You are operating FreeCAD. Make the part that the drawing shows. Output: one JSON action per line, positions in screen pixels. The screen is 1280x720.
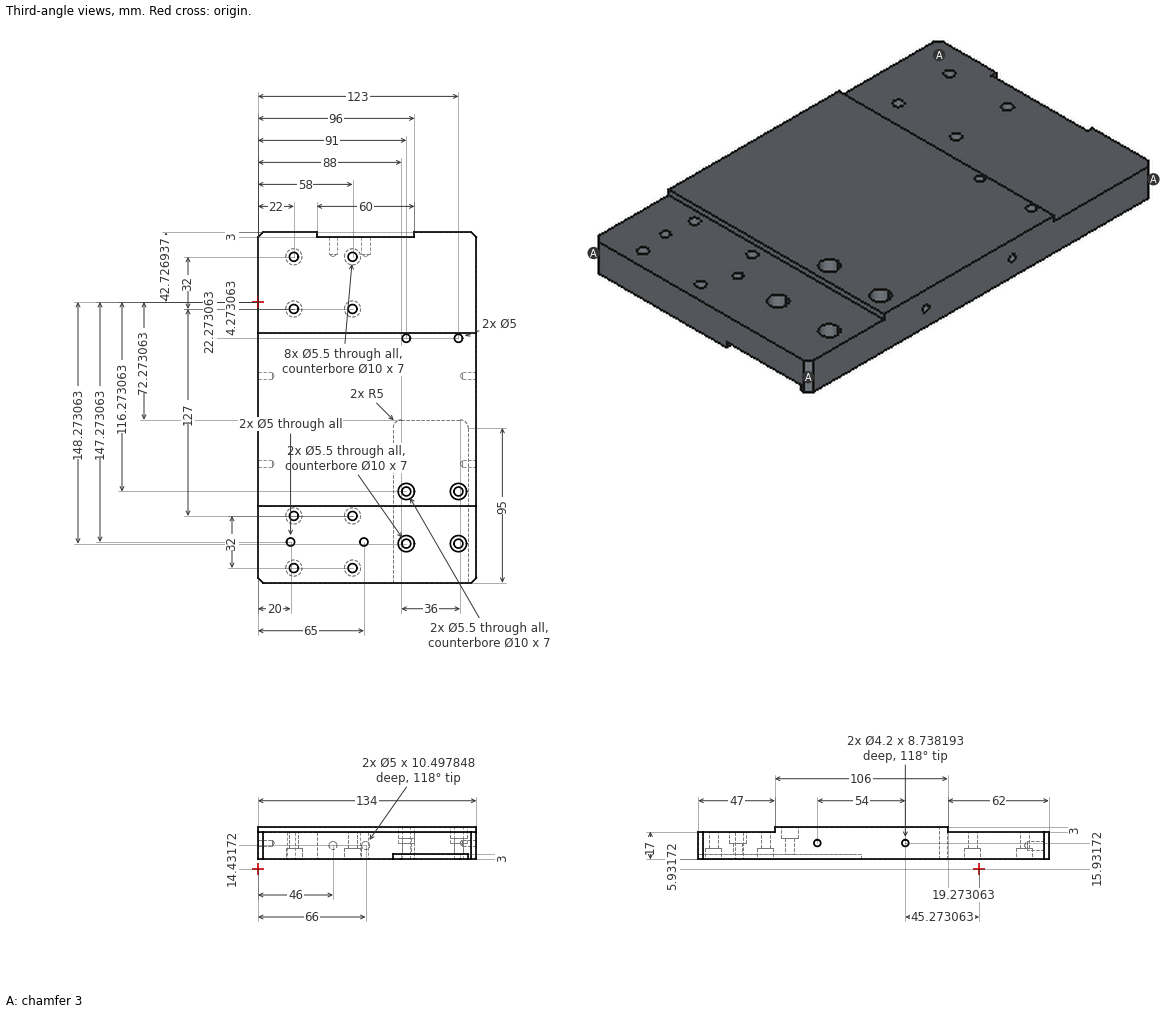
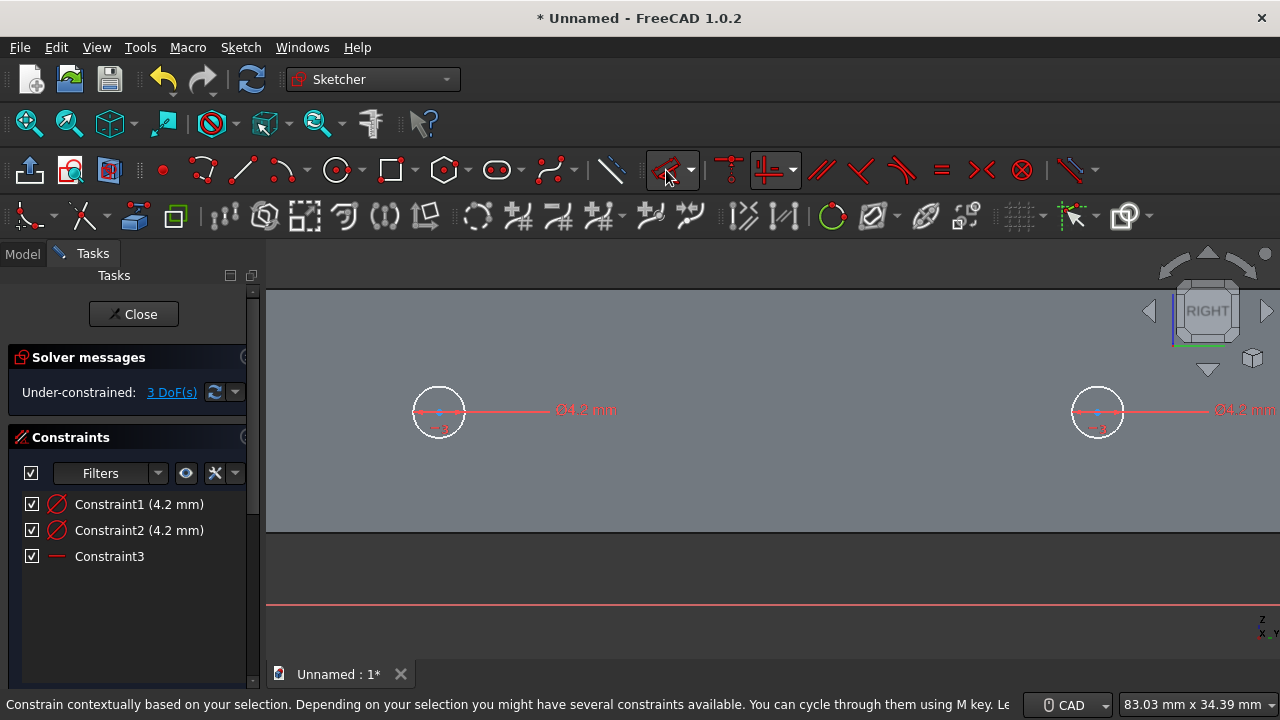
{"action": "left_click", "coordinate": [1098, 412]}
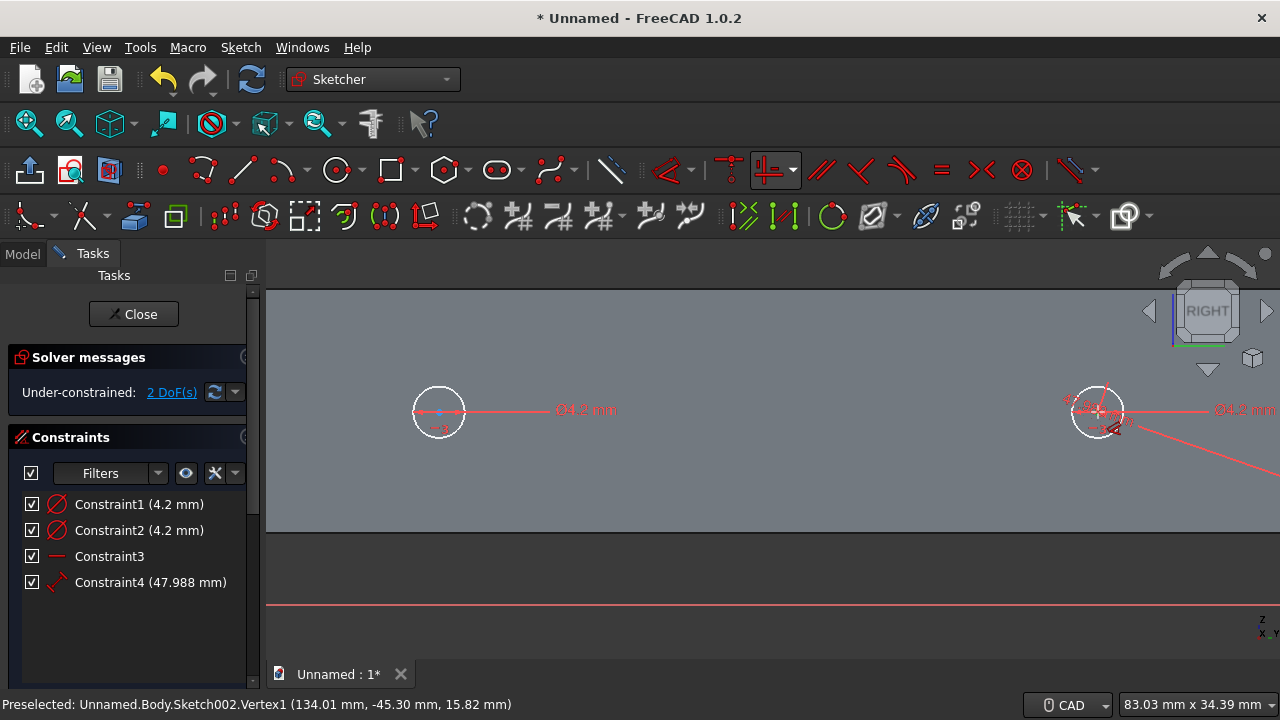
{"action": "left_click", "coordinate": [439, 412]}
{"action": "left_click", "coordinate": [768, 378]}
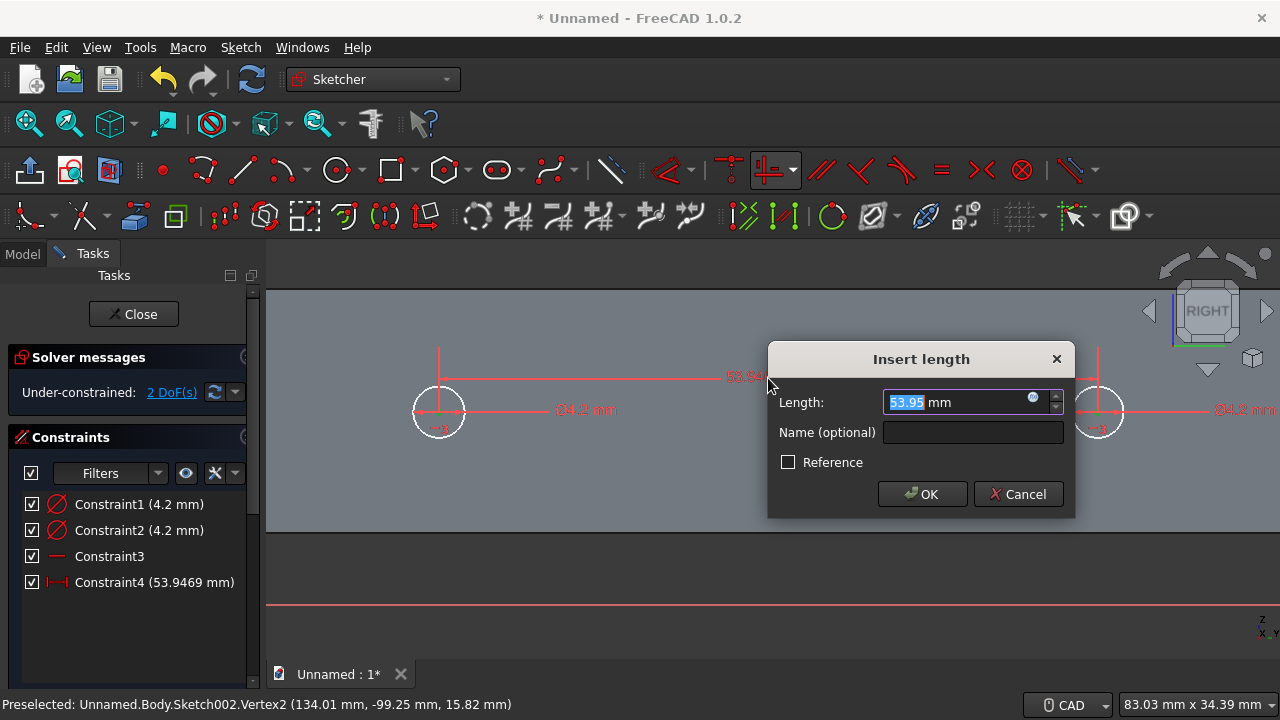
{"action": "type", "text": "54"}
{"action": "key", "text": "Return"}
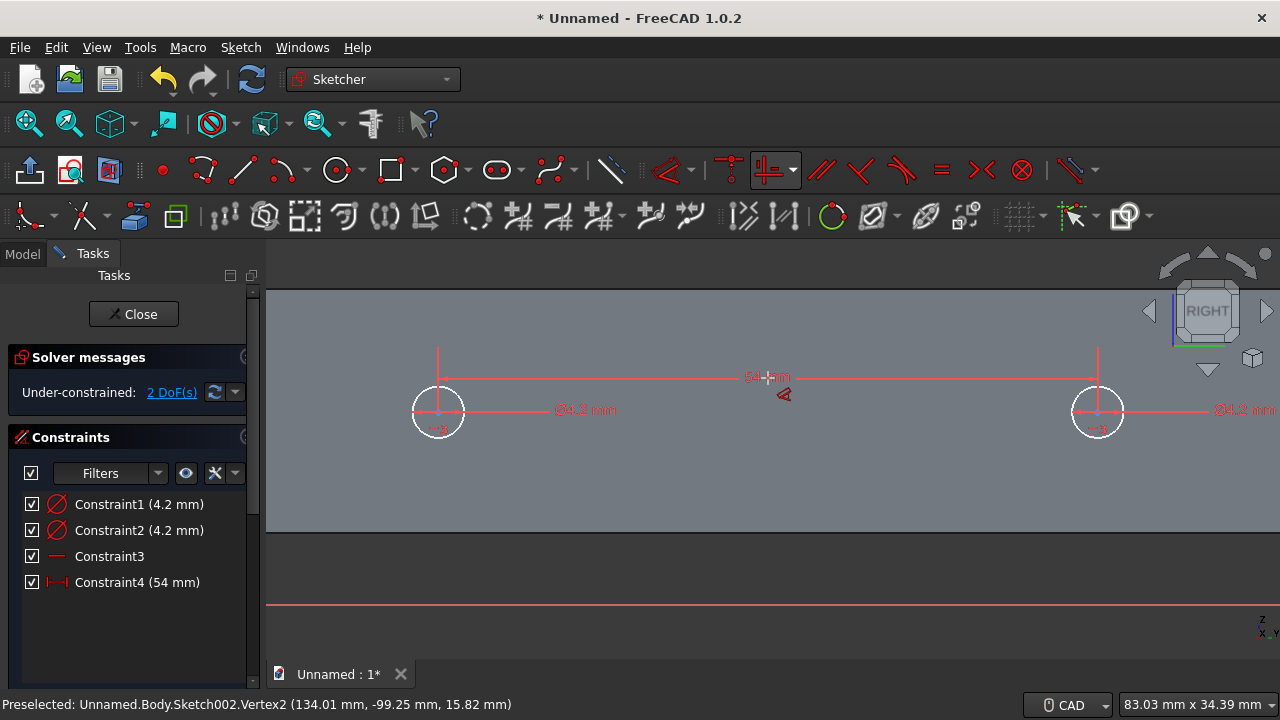
{"action": "left_click", "coordinate": [1098, 412]}
{"action": "left_click", "coordinate": [1064, 509]}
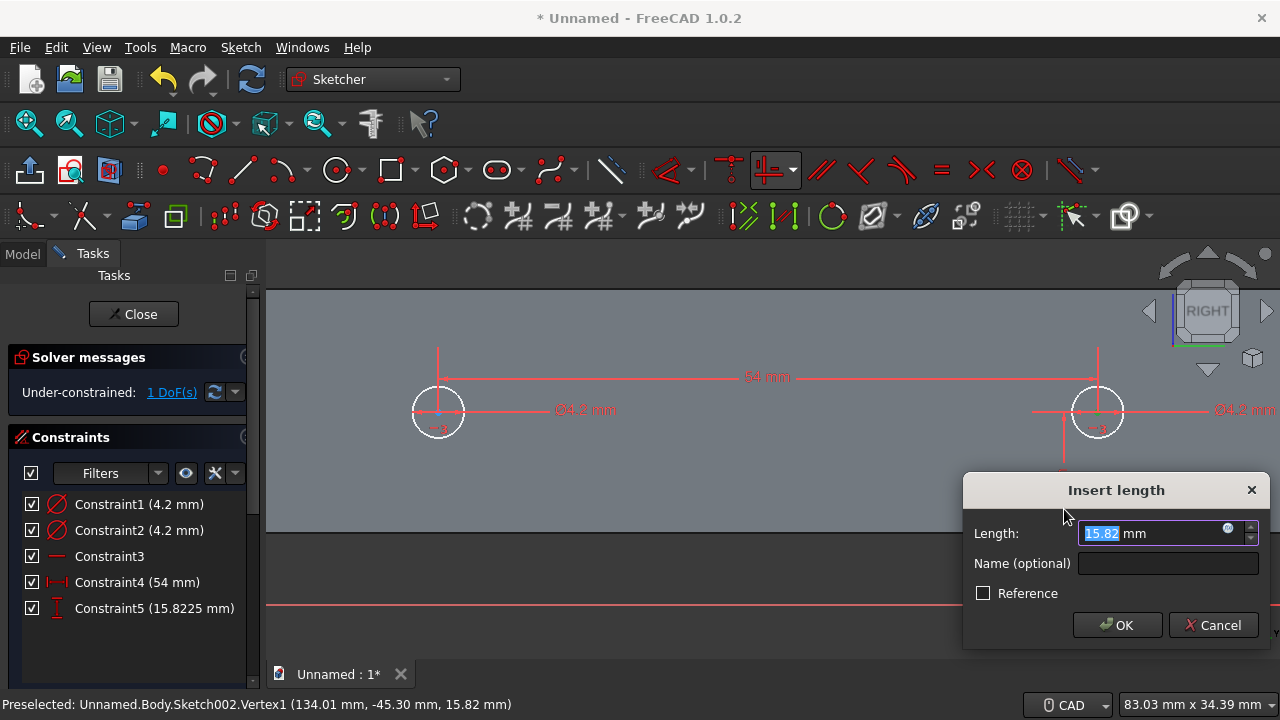
{"action": "type", "text": "15.93172"}
{"action": "key", "text": "Return"}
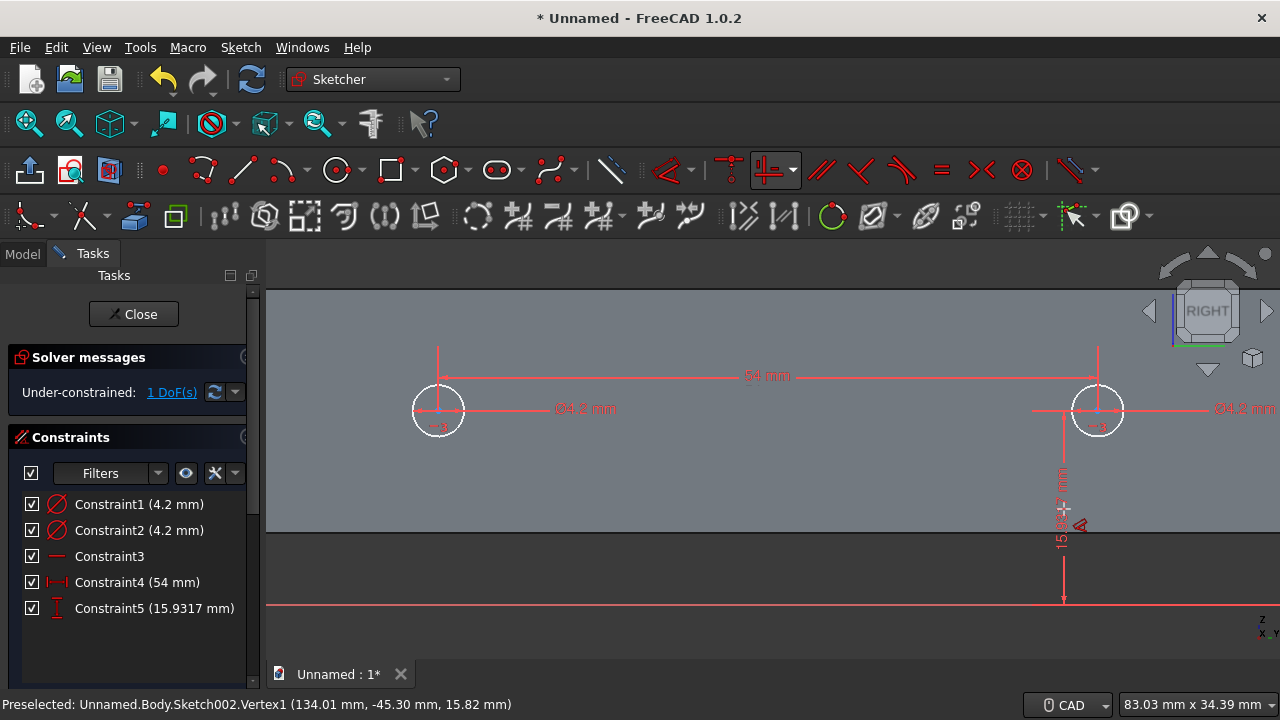
{"action": "left_click", "coordinate": [1098, 411]}
{"action": "left_click", "coordinate": [1106, 353]}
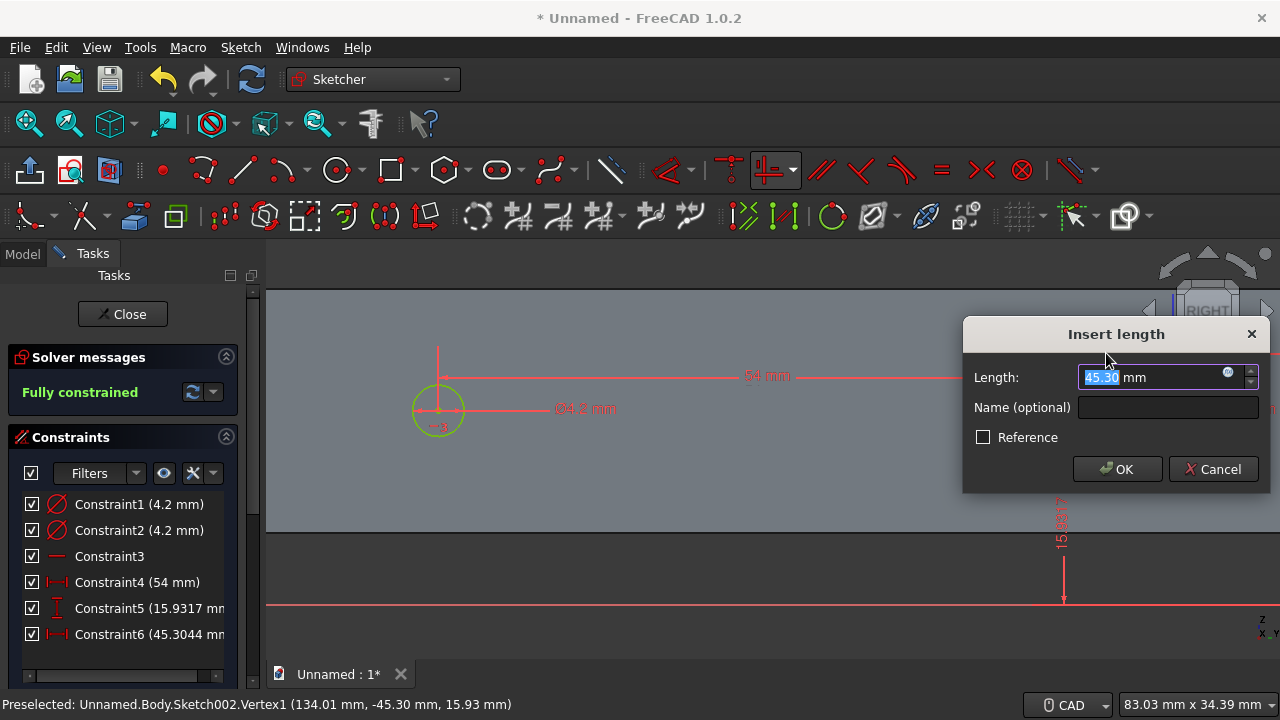
{"action": "type", "text": "45.273063"}
{"action": "key", "text": "Return"}
{"action": "key", "text": "Escape"}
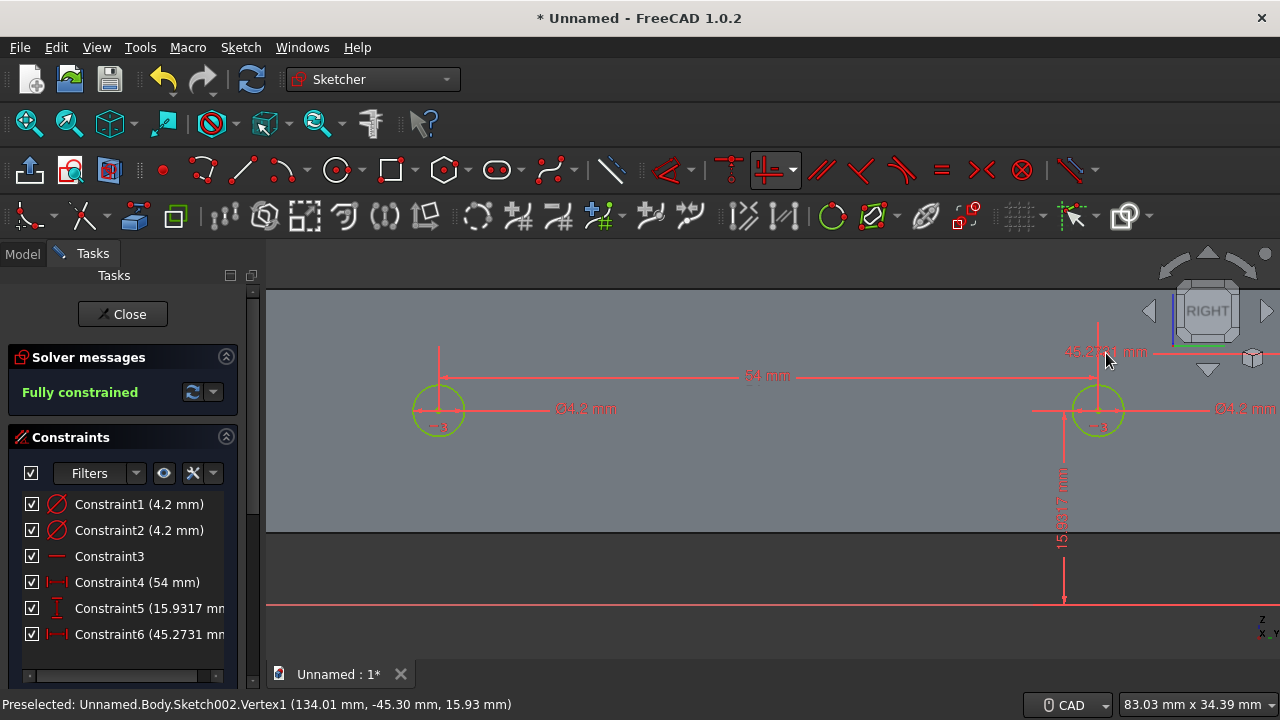
{"action": "left_click", "coordinate": [123, 314]}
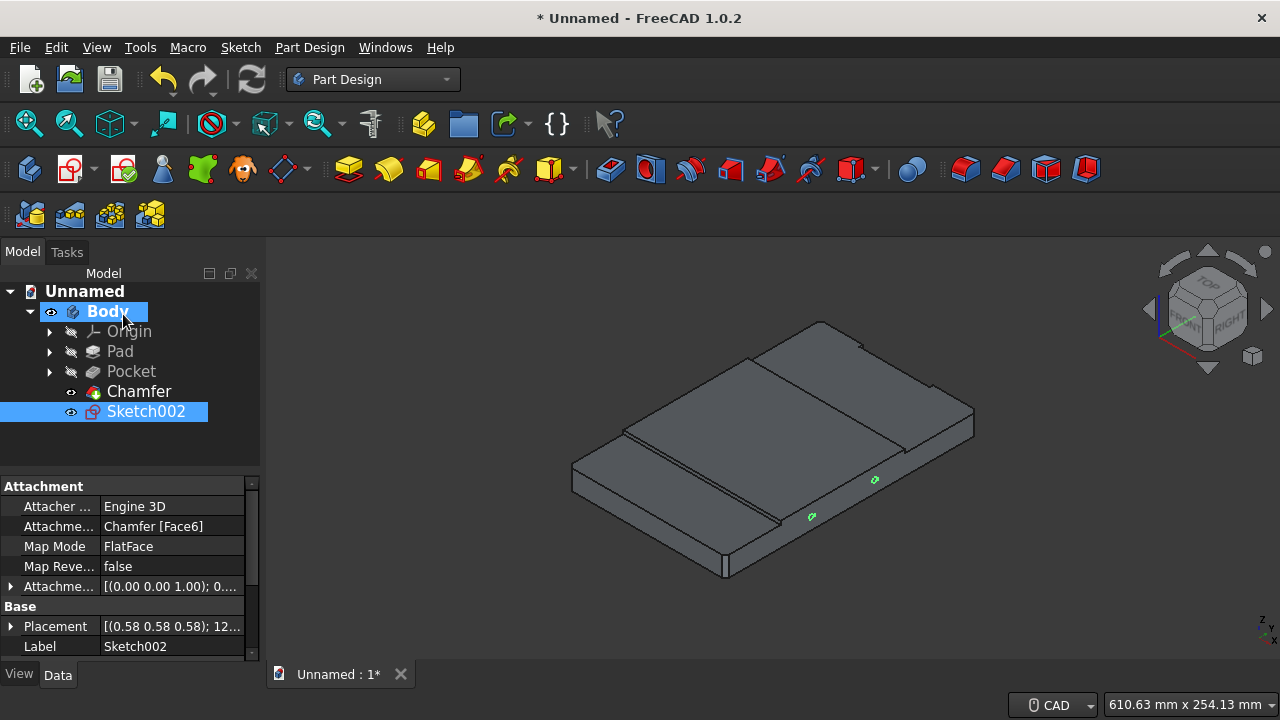
{"action": "left_click", "coordinate": [652, 170]}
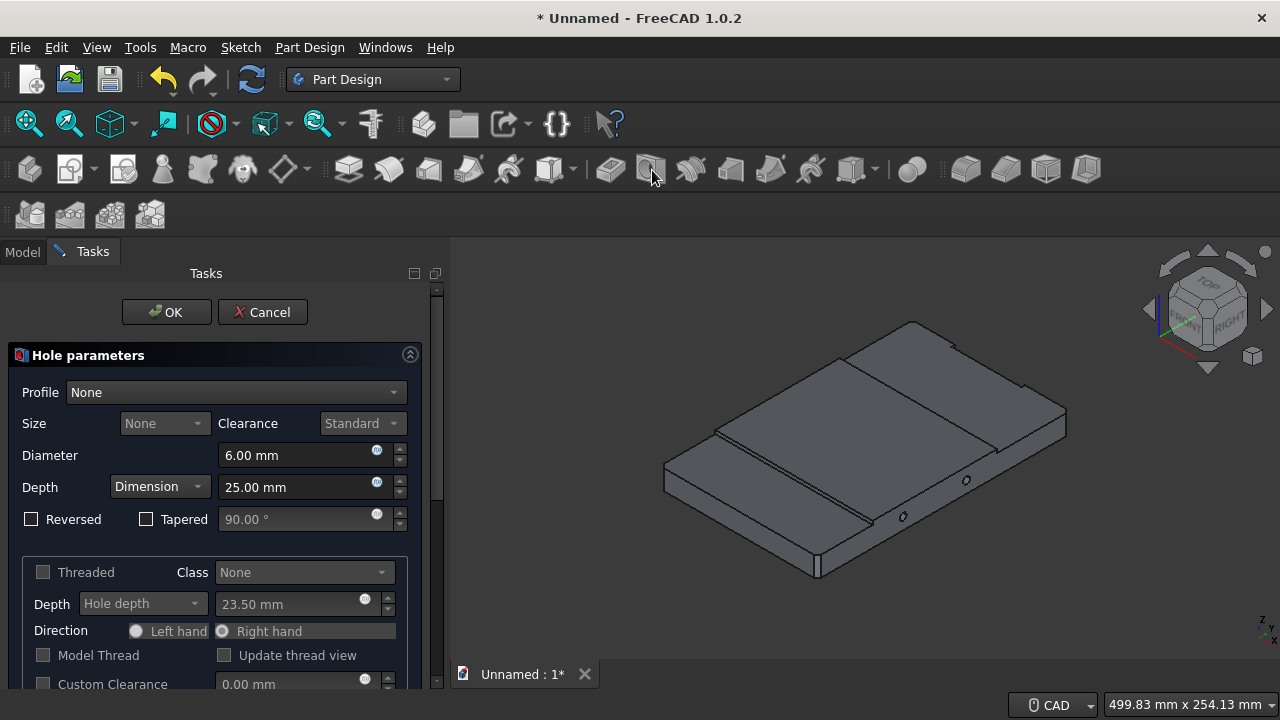
{"action": "triple_click", "coordinate": [305, 455]}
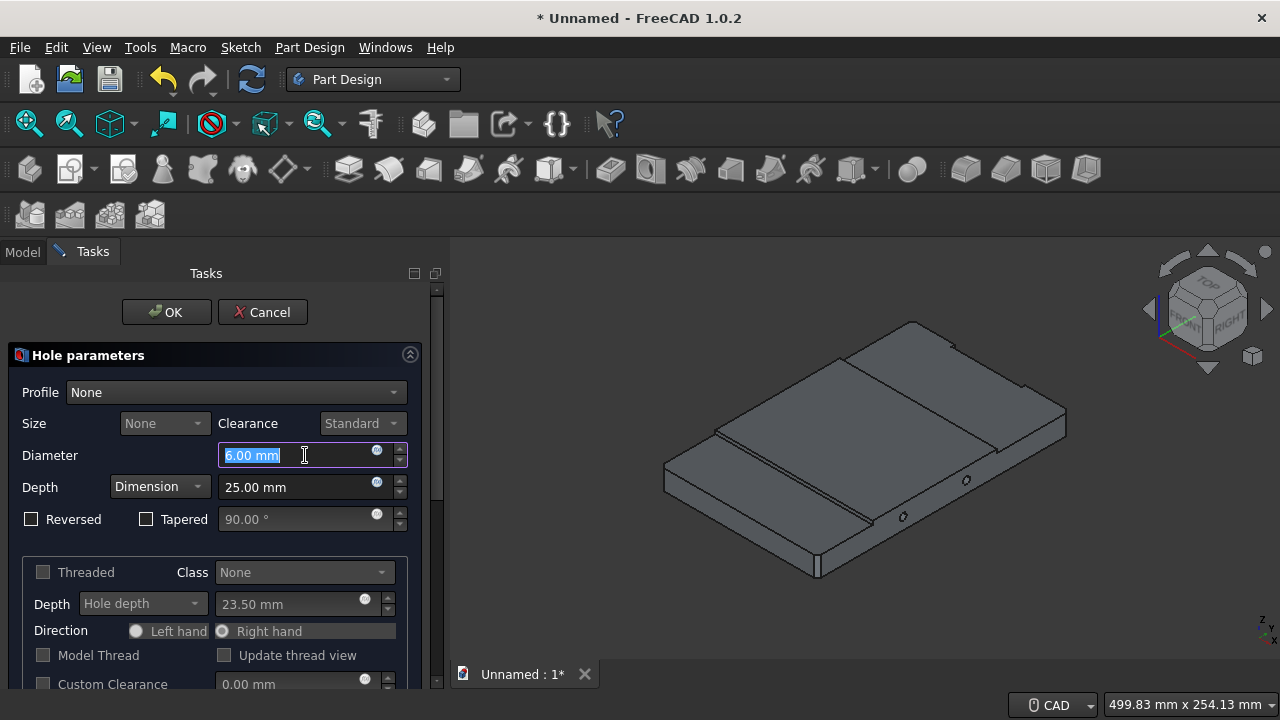
{"action": "type", "text": "4.2"}
{"action": "key", "text": "Tab"}